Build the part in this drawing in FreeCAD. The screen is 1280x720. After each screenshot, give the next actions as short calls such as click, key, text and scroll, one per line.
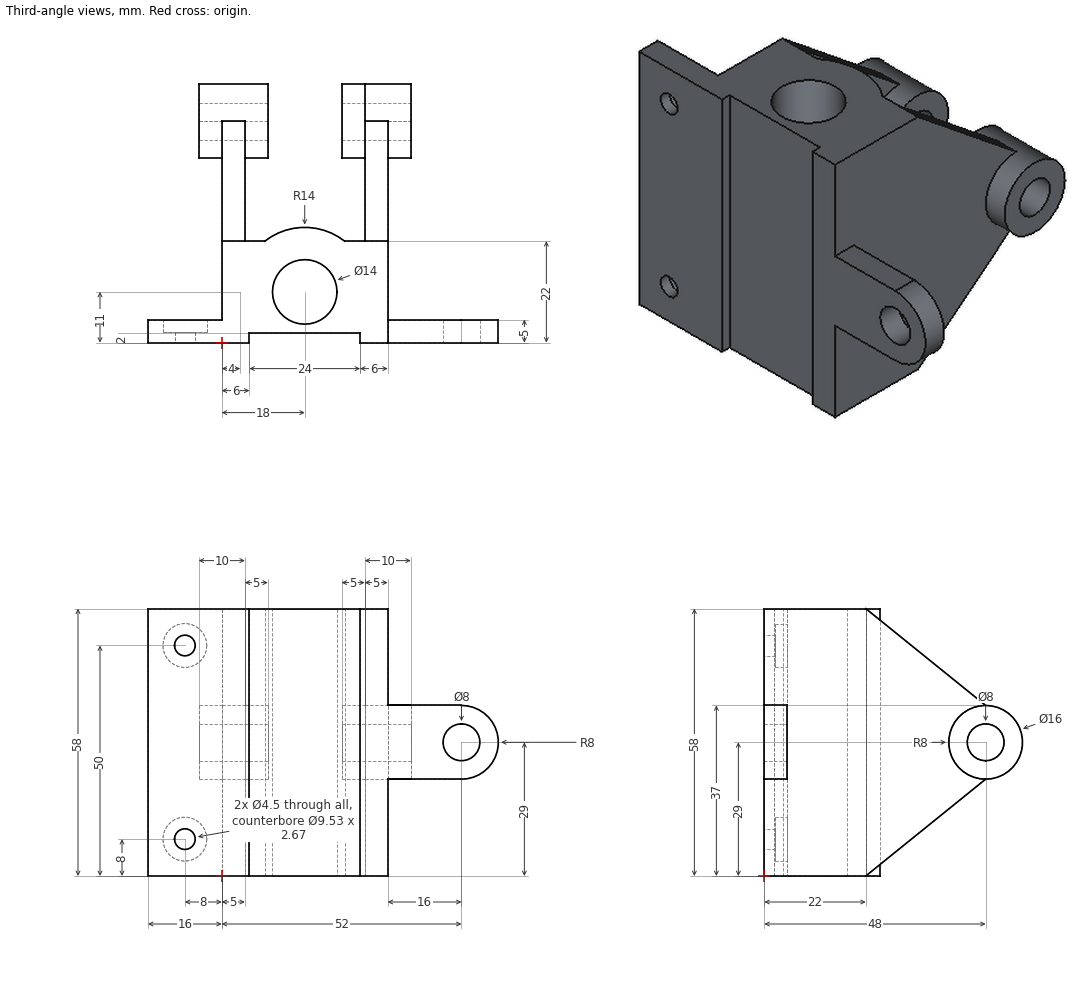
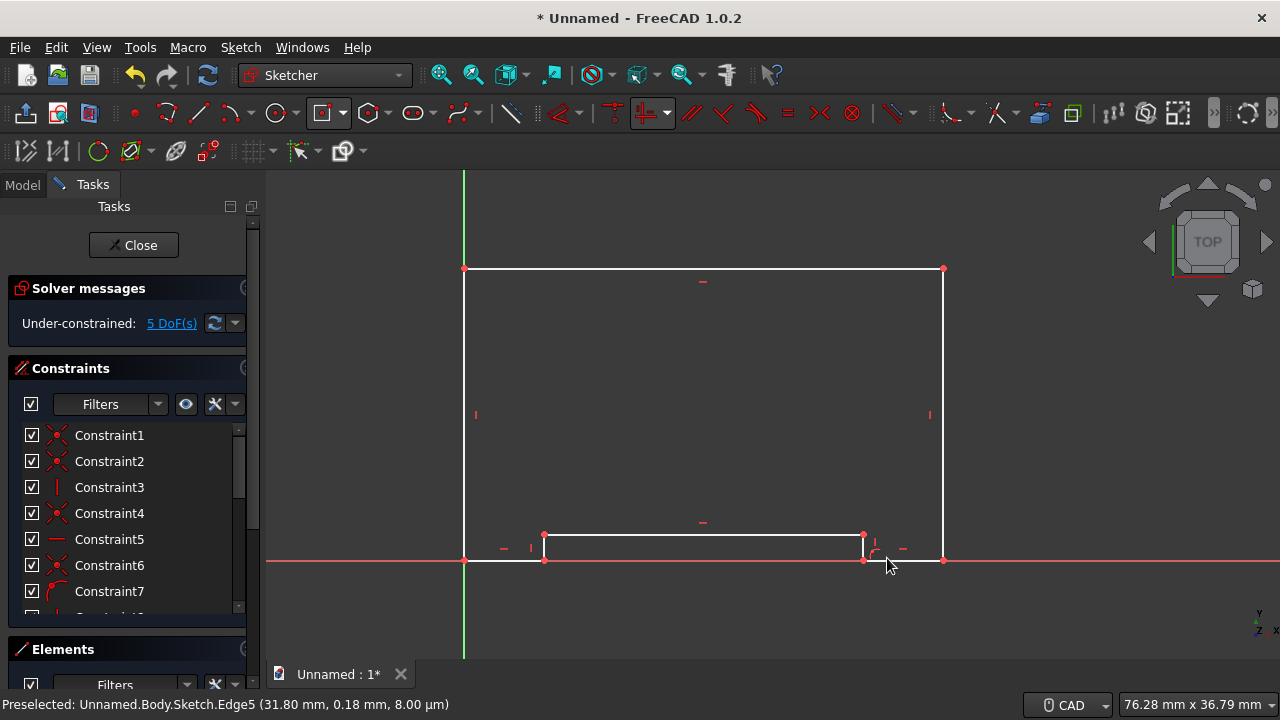
key(d)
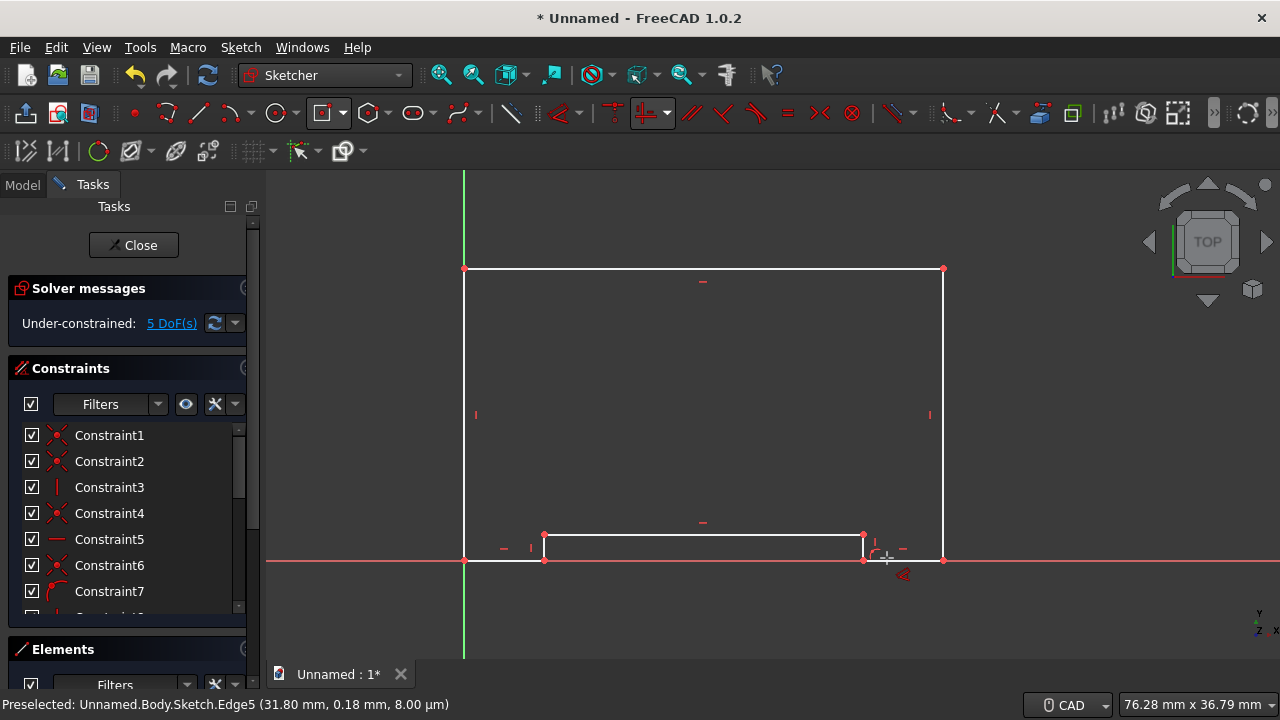
click(488, 561)
click(504, 595)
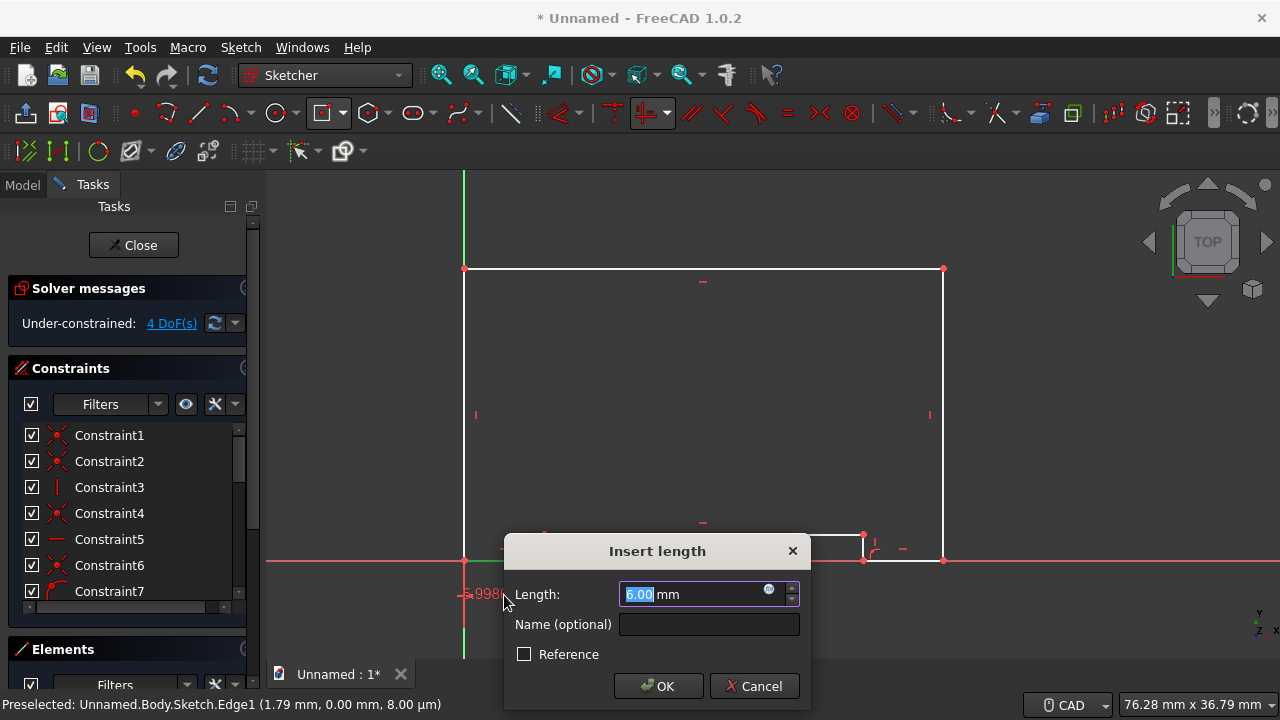
text(6)
key(Return)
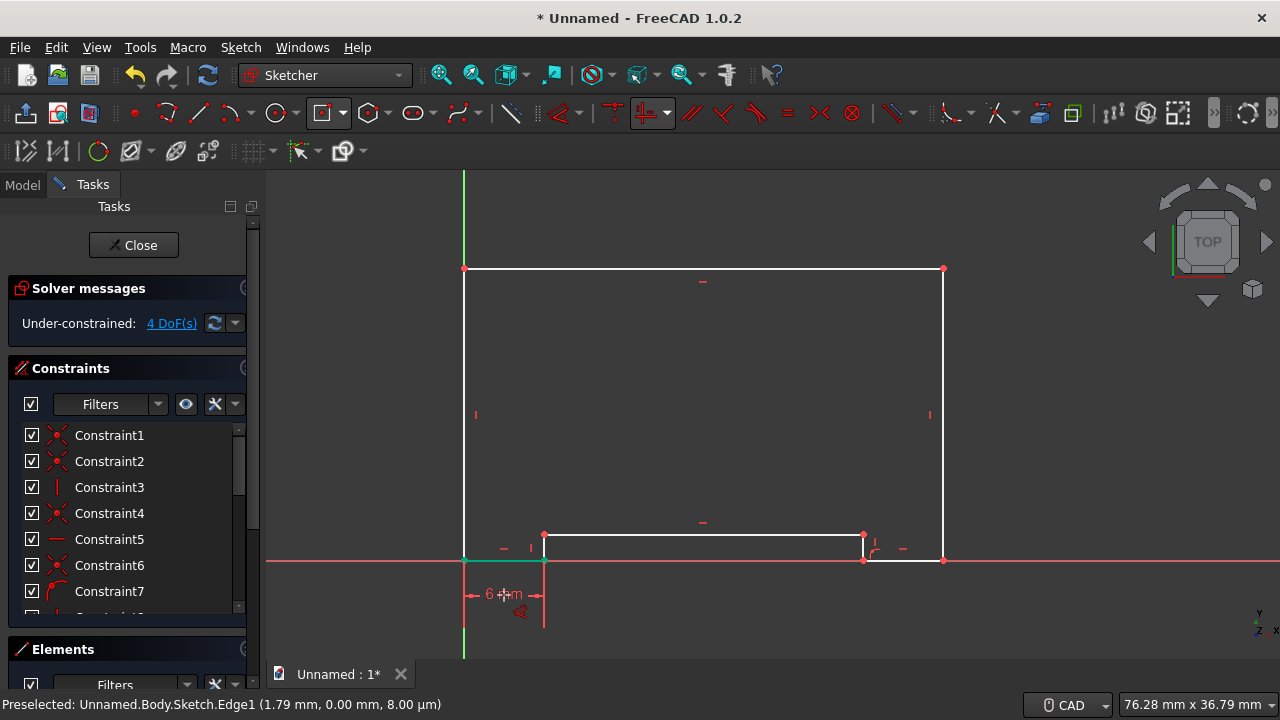
scroll(544, 551, up, 3)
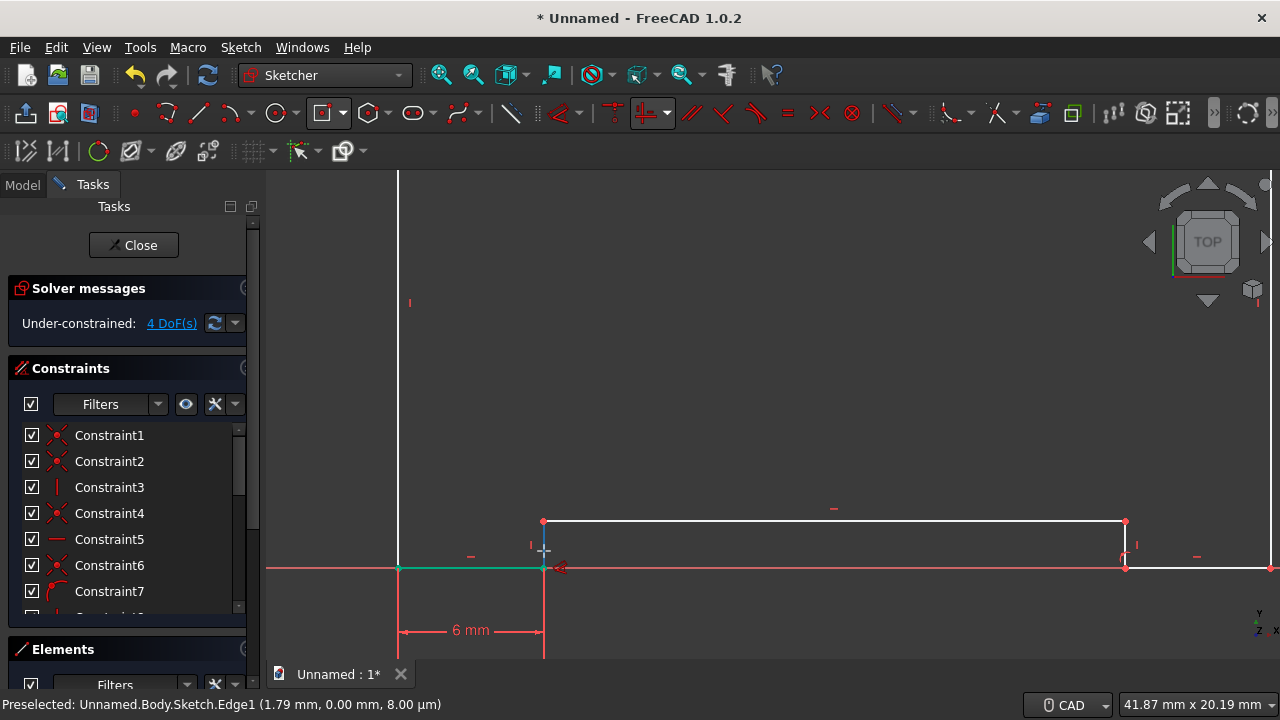
click(544, 549)
click(510, 545)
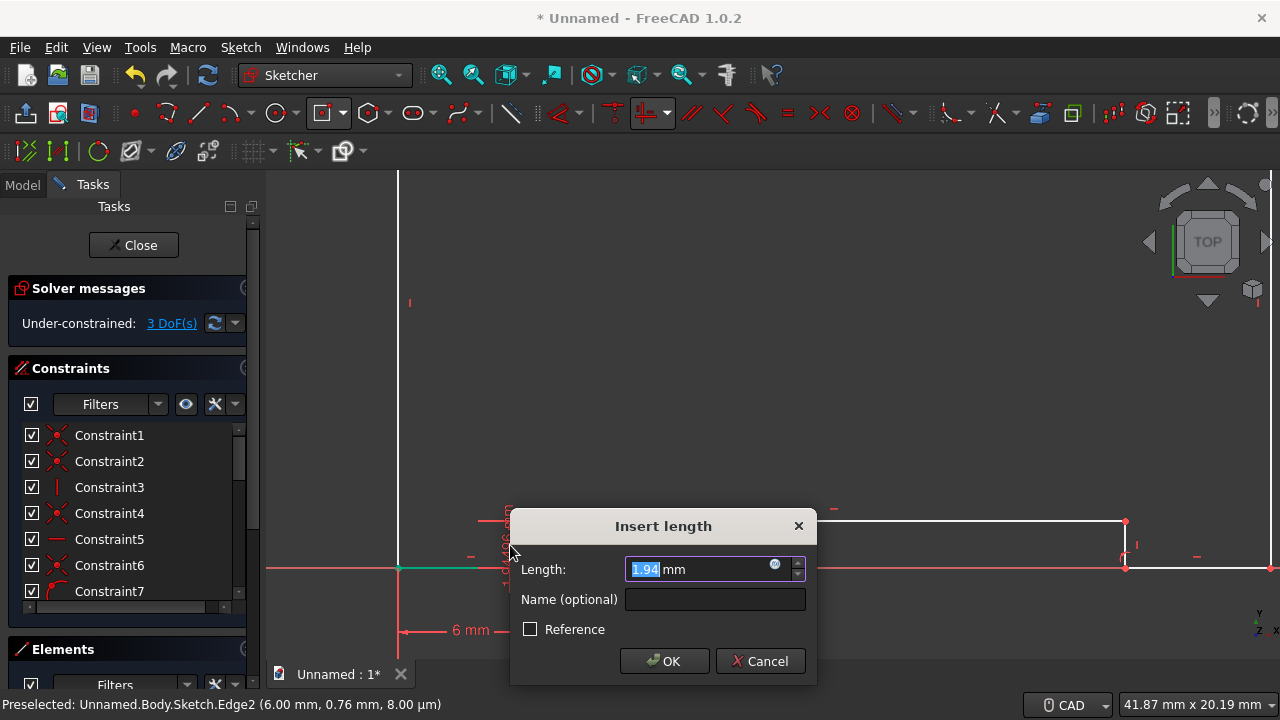
text(2)
key(Return)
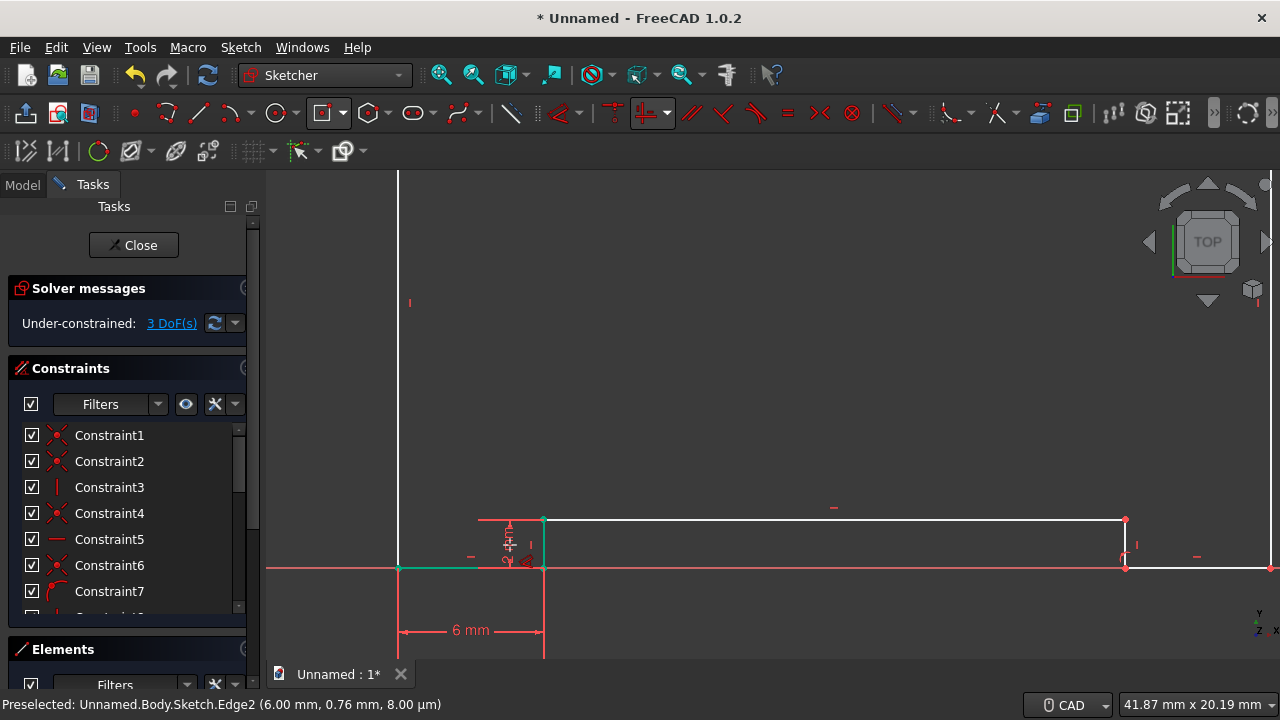
scroll(546, 551, down, 3)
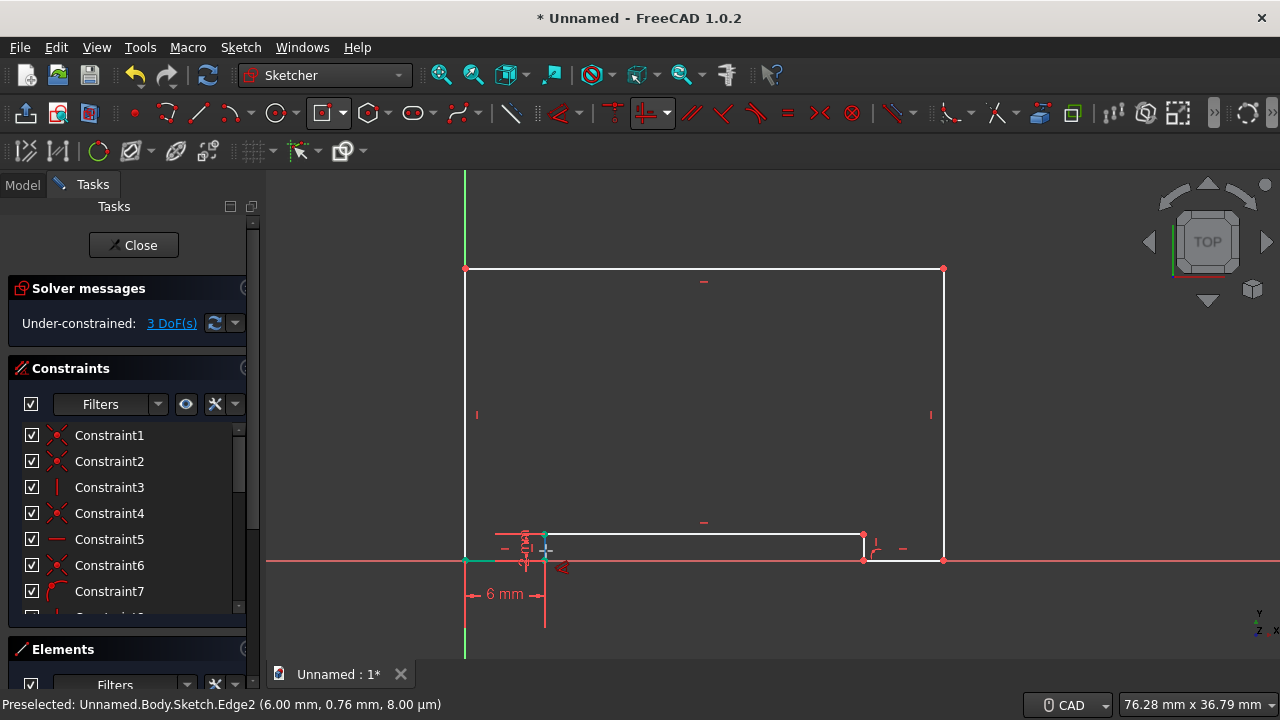
click(888, 561)
click(904, 595)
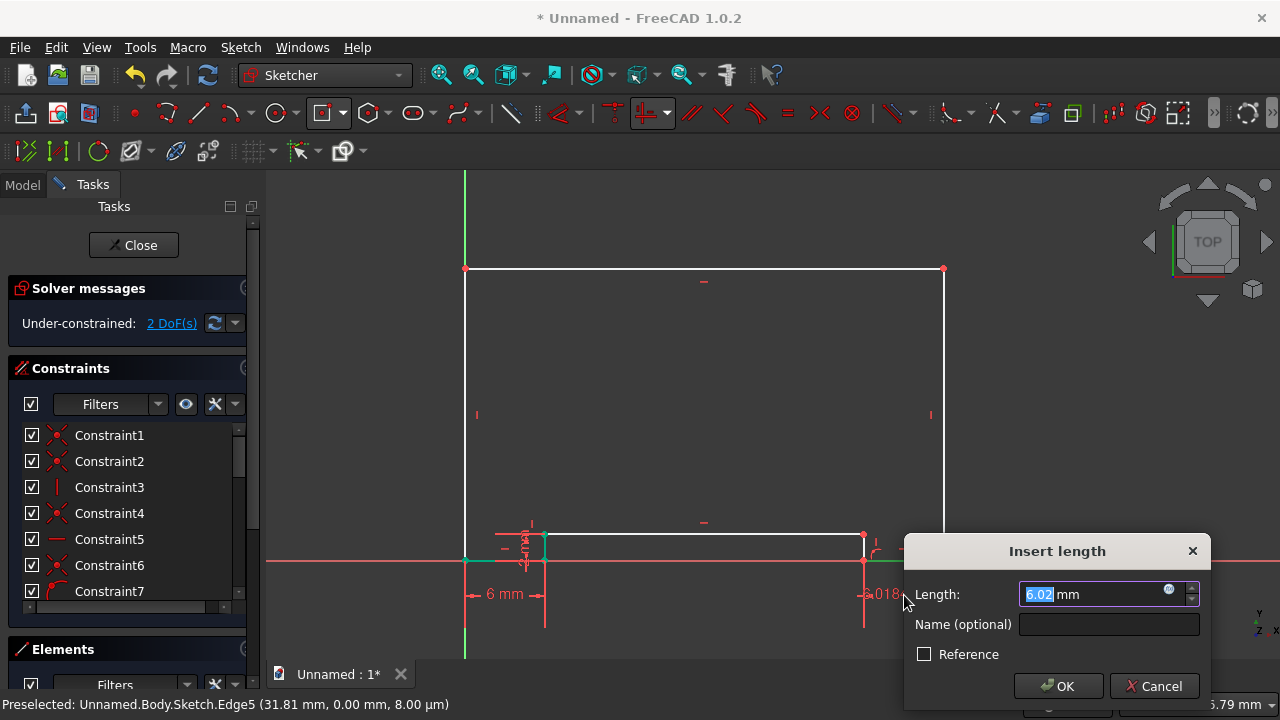
text(6)
key(Return)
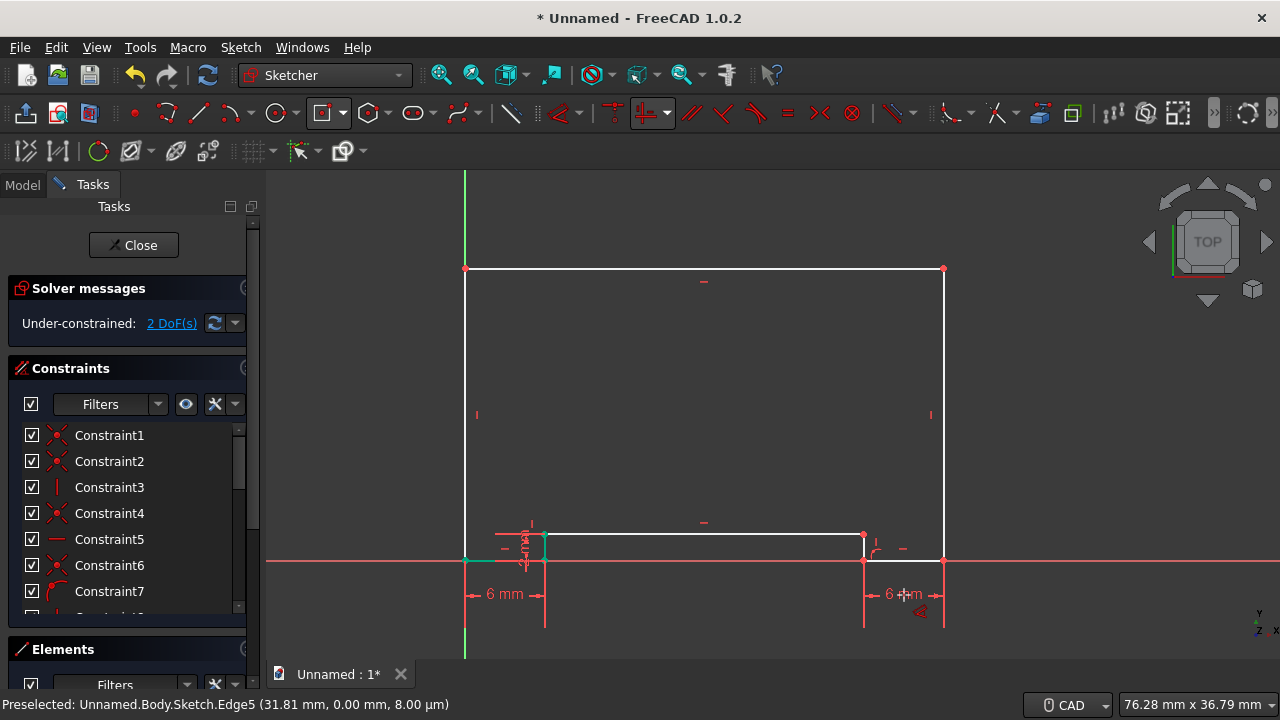
click(641, 534)
click(704, 500)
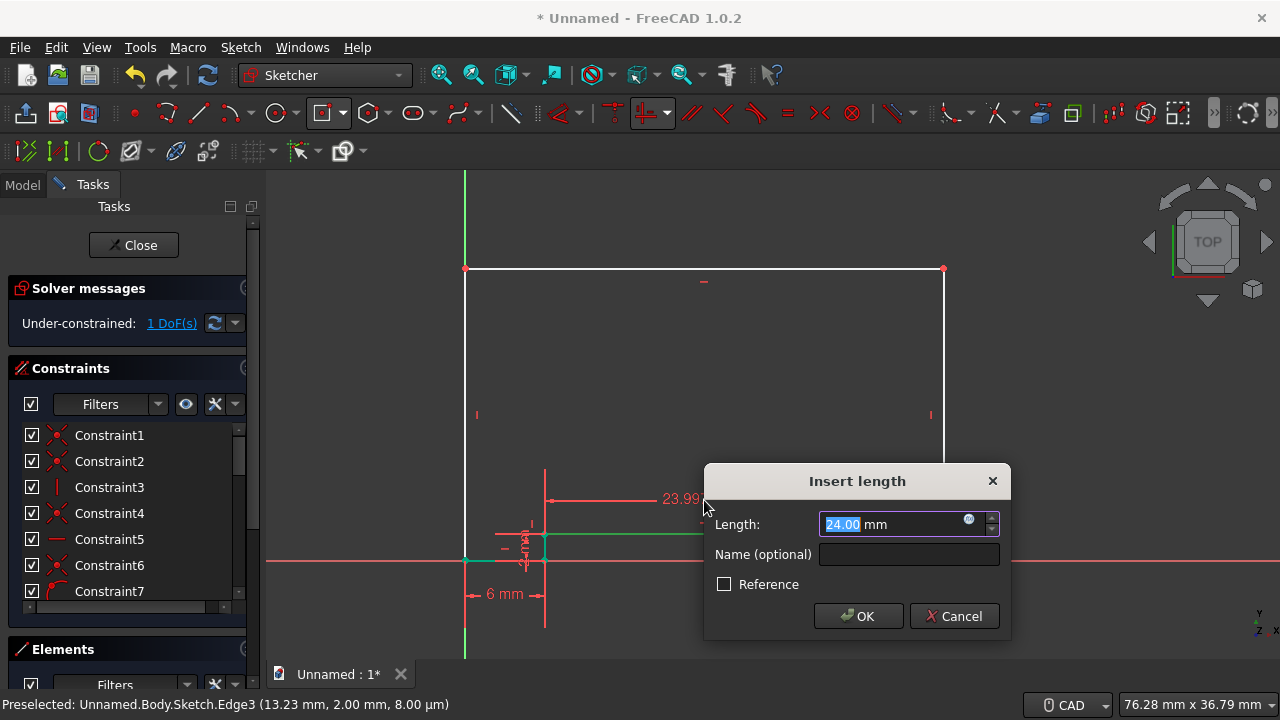
text(24)
key(Return)